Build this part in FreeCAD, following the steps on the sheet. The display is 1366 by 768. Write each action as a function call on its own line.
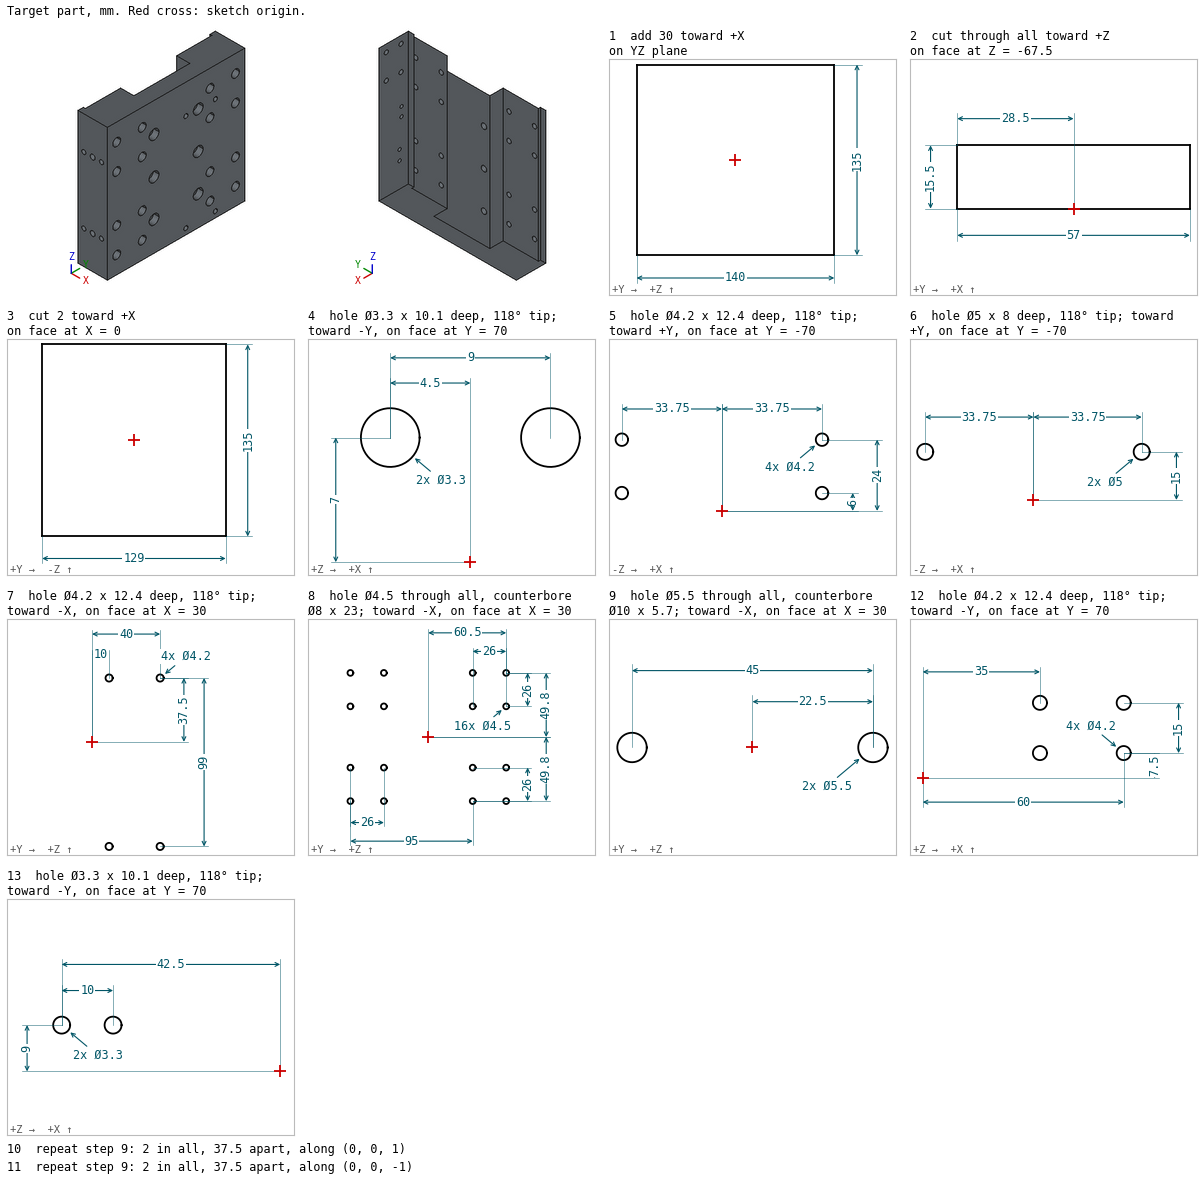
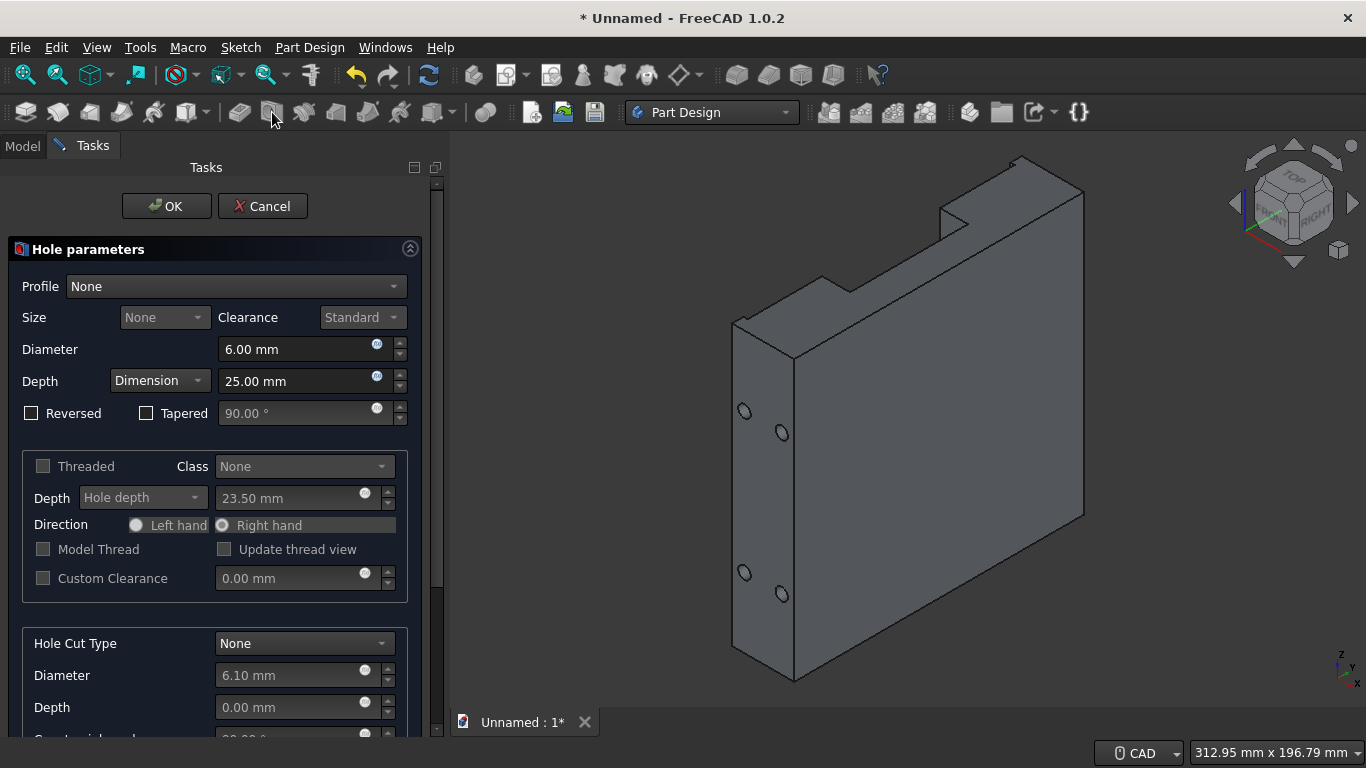
triple_click(305, 349)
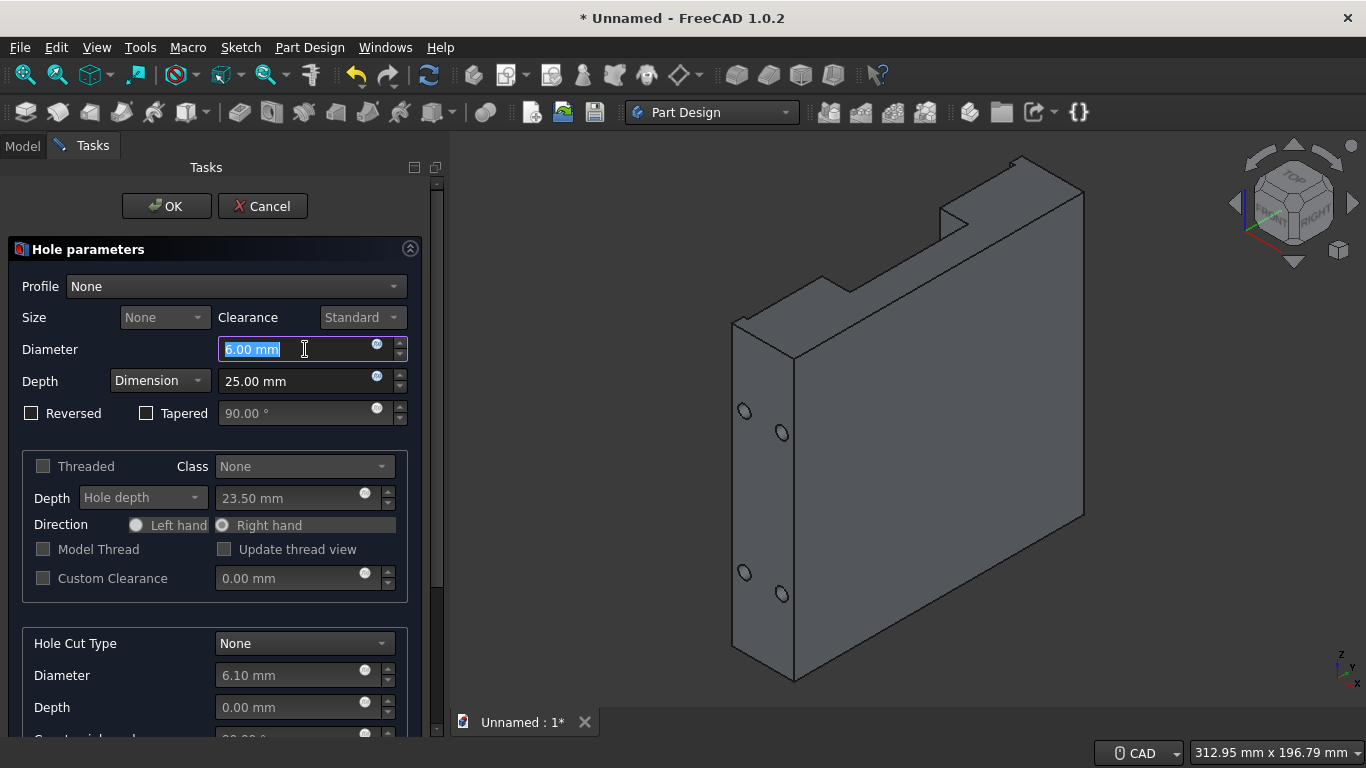
text(4.2)
key(Tab)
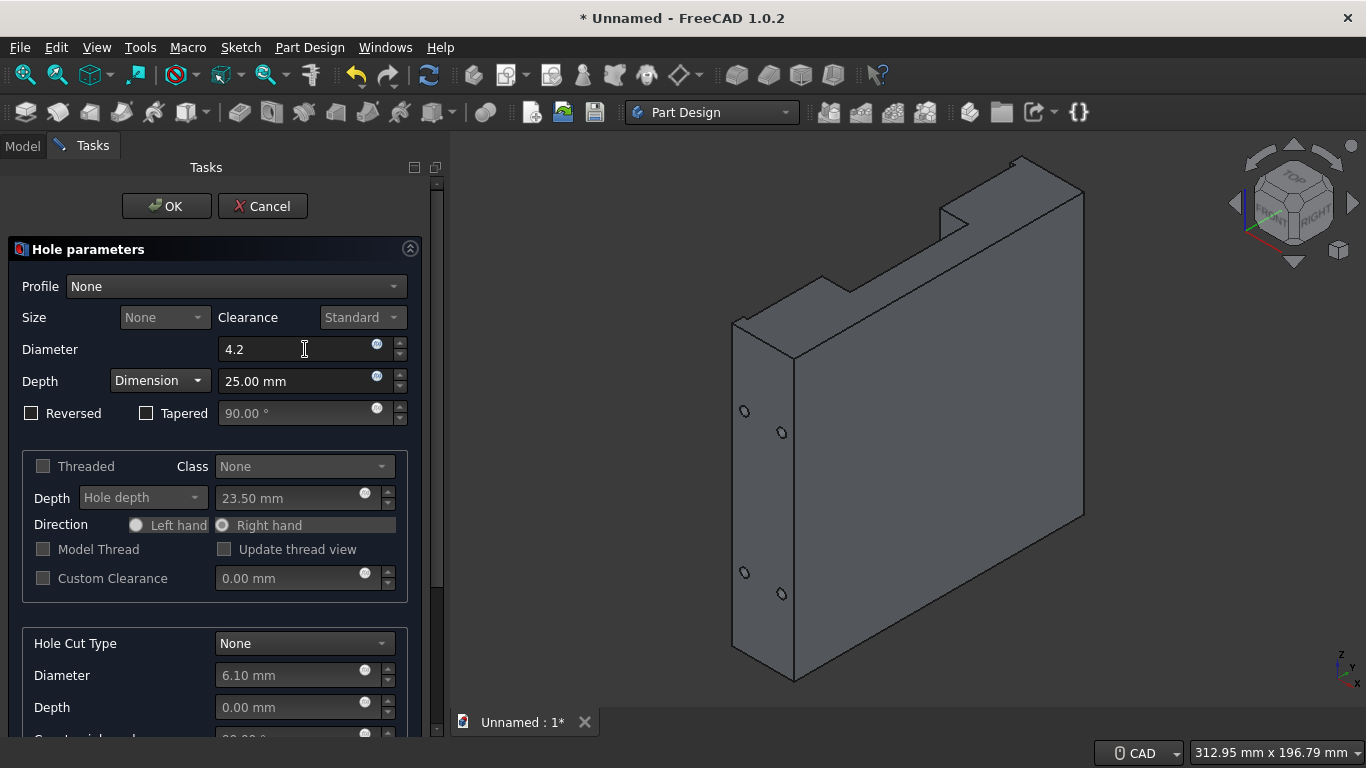
triple_click(305, 381)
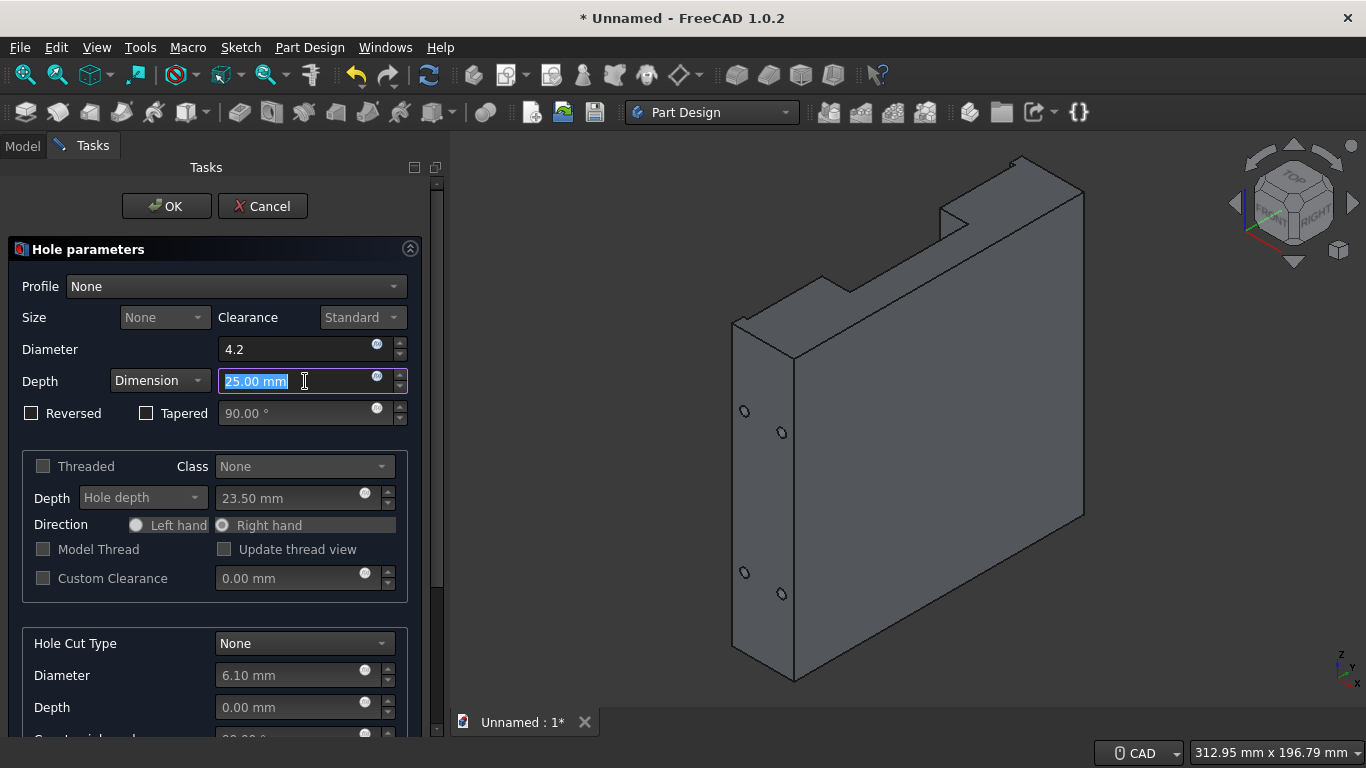
text(12.4)
key(Tab)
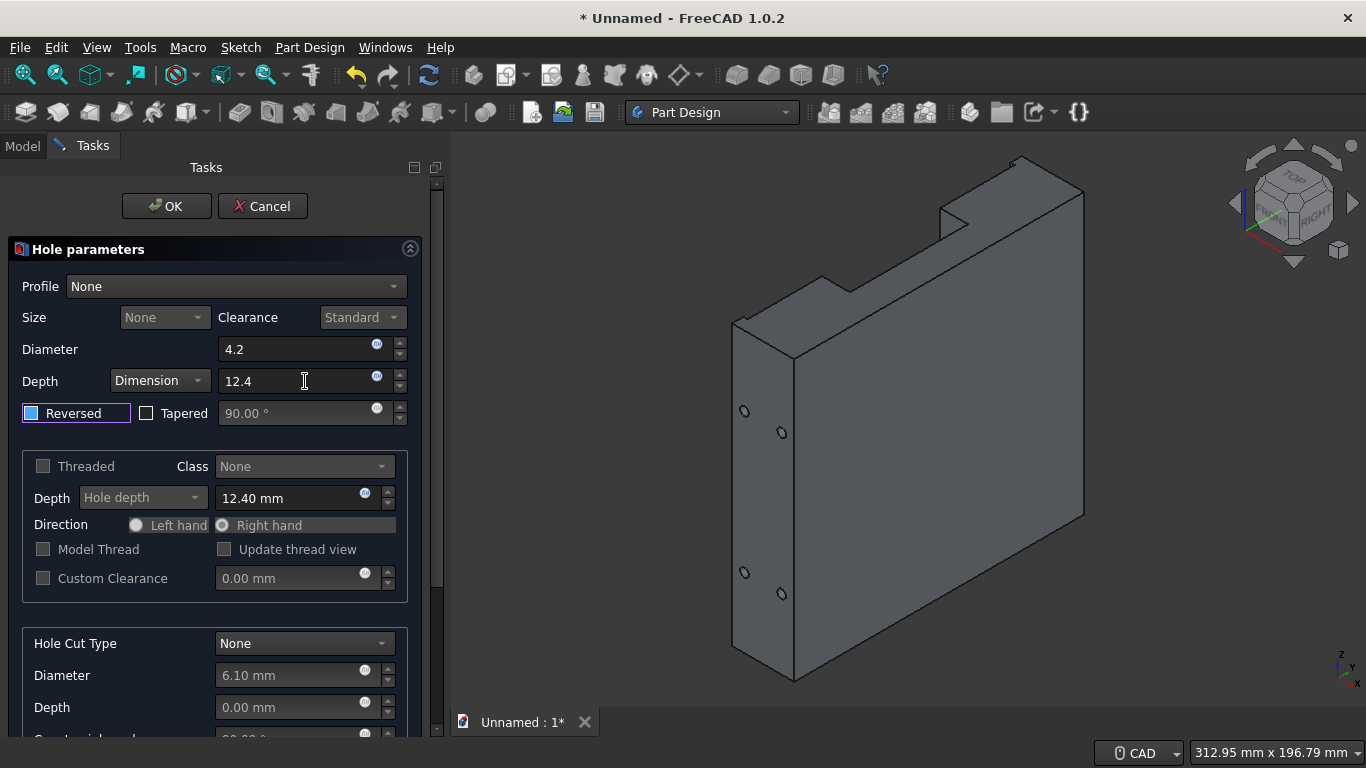
click(167, 206)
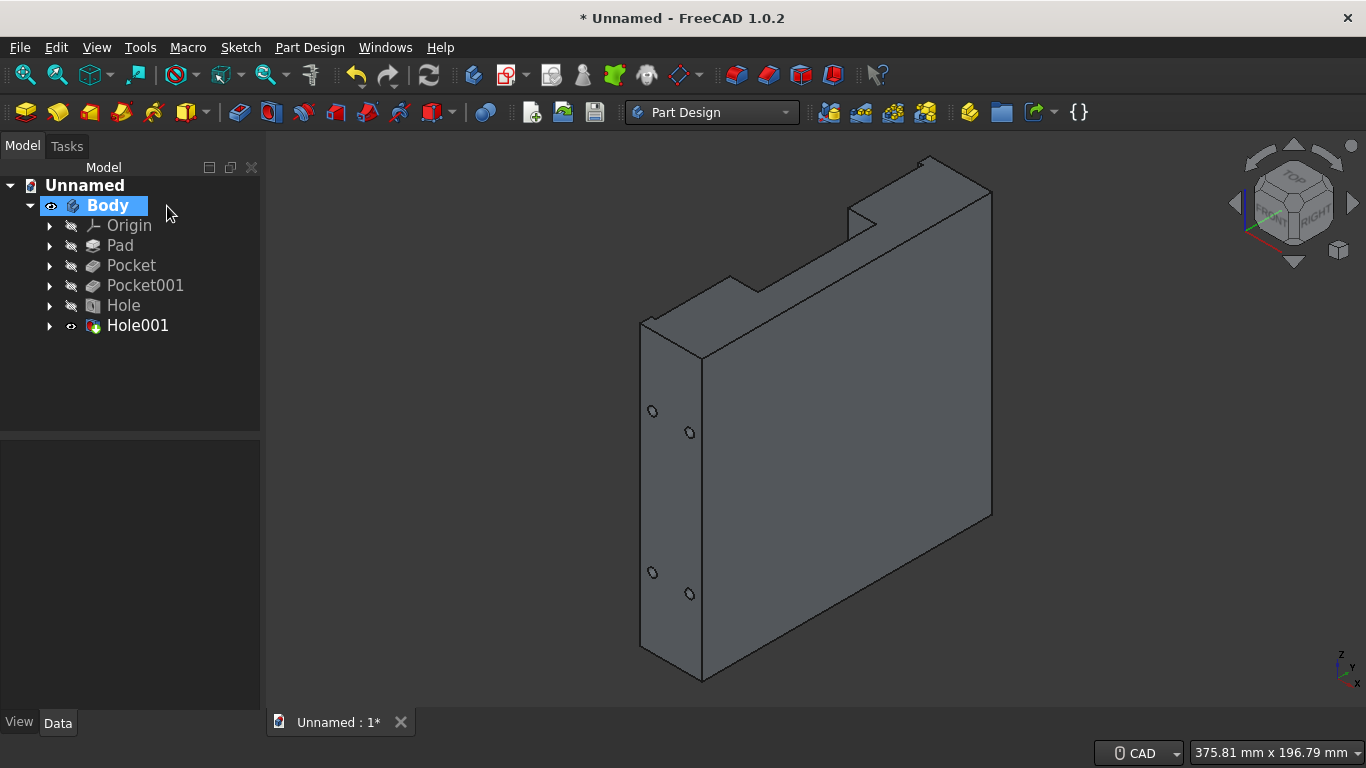
click(671, 502)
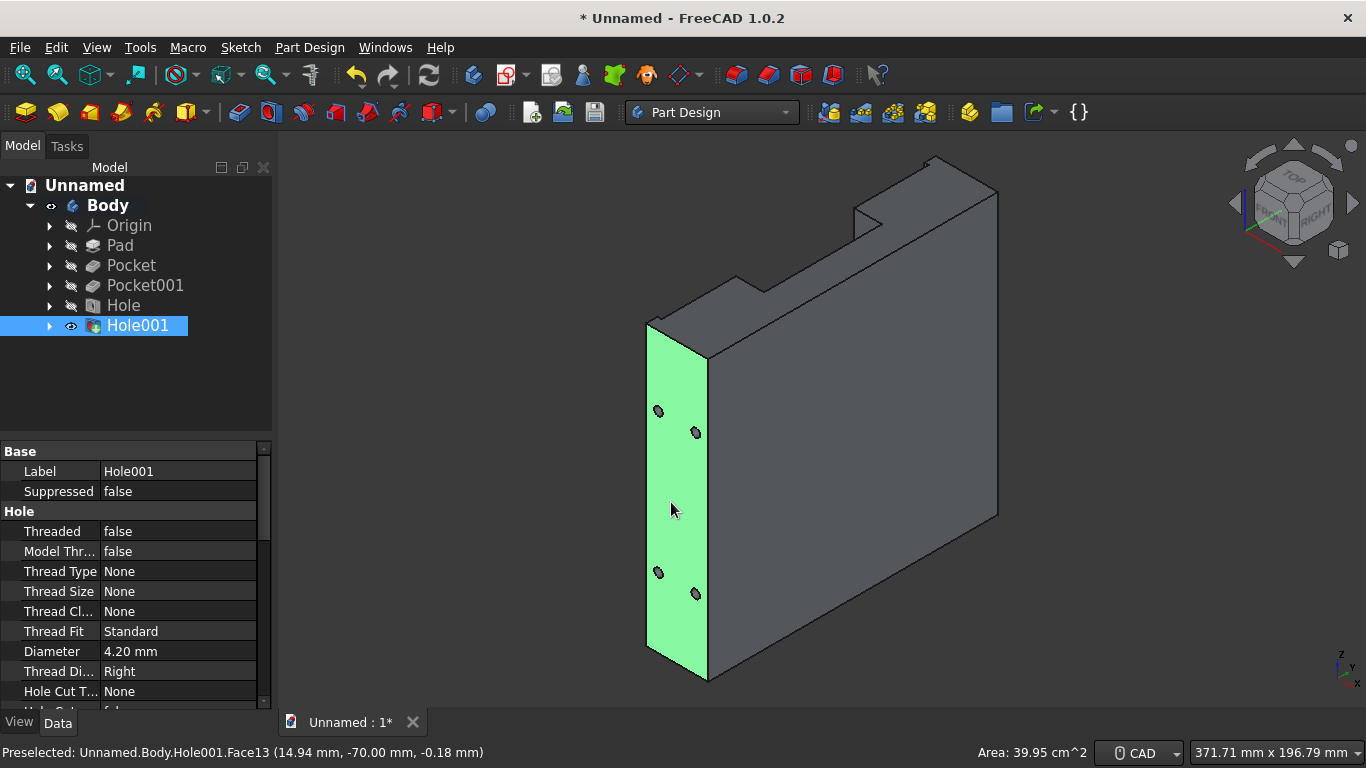
click(506, 76)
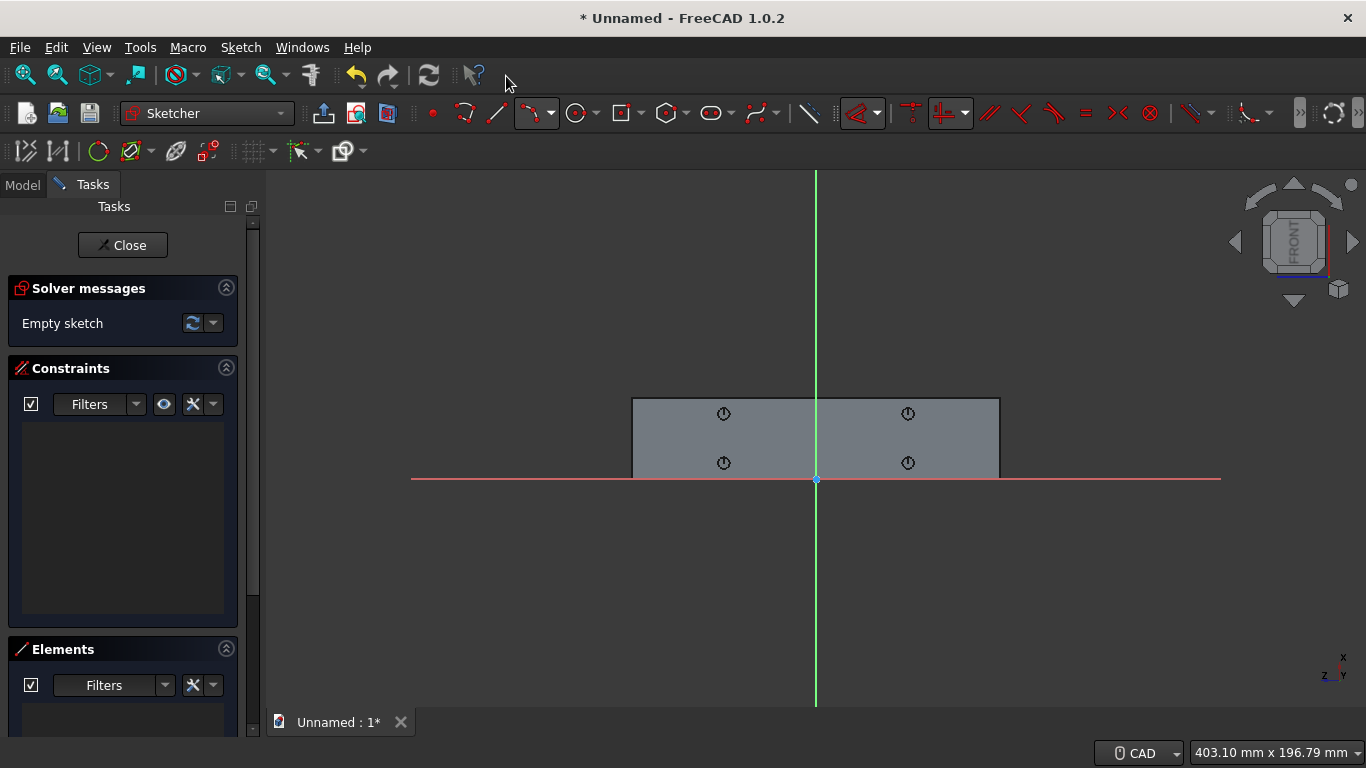
scroll(846, 463, up, 6)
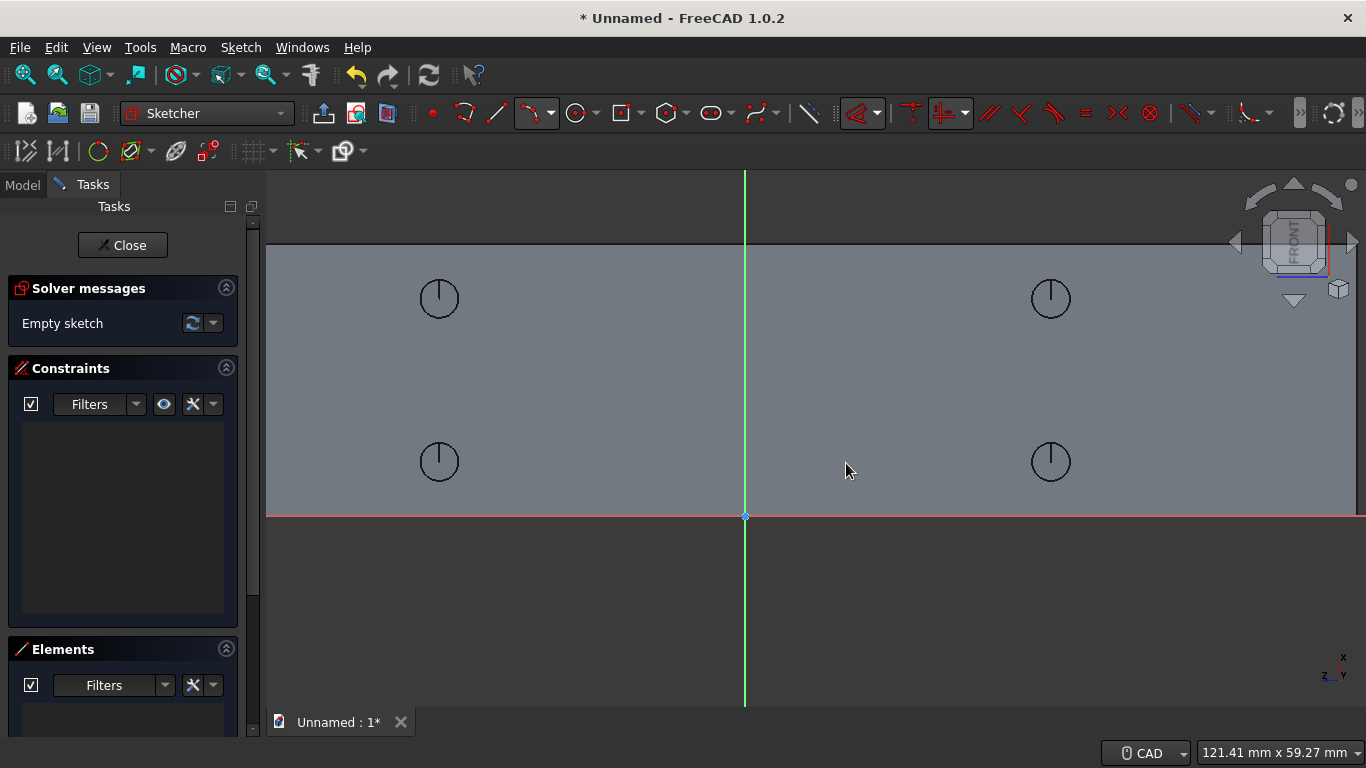
click(576, 114)